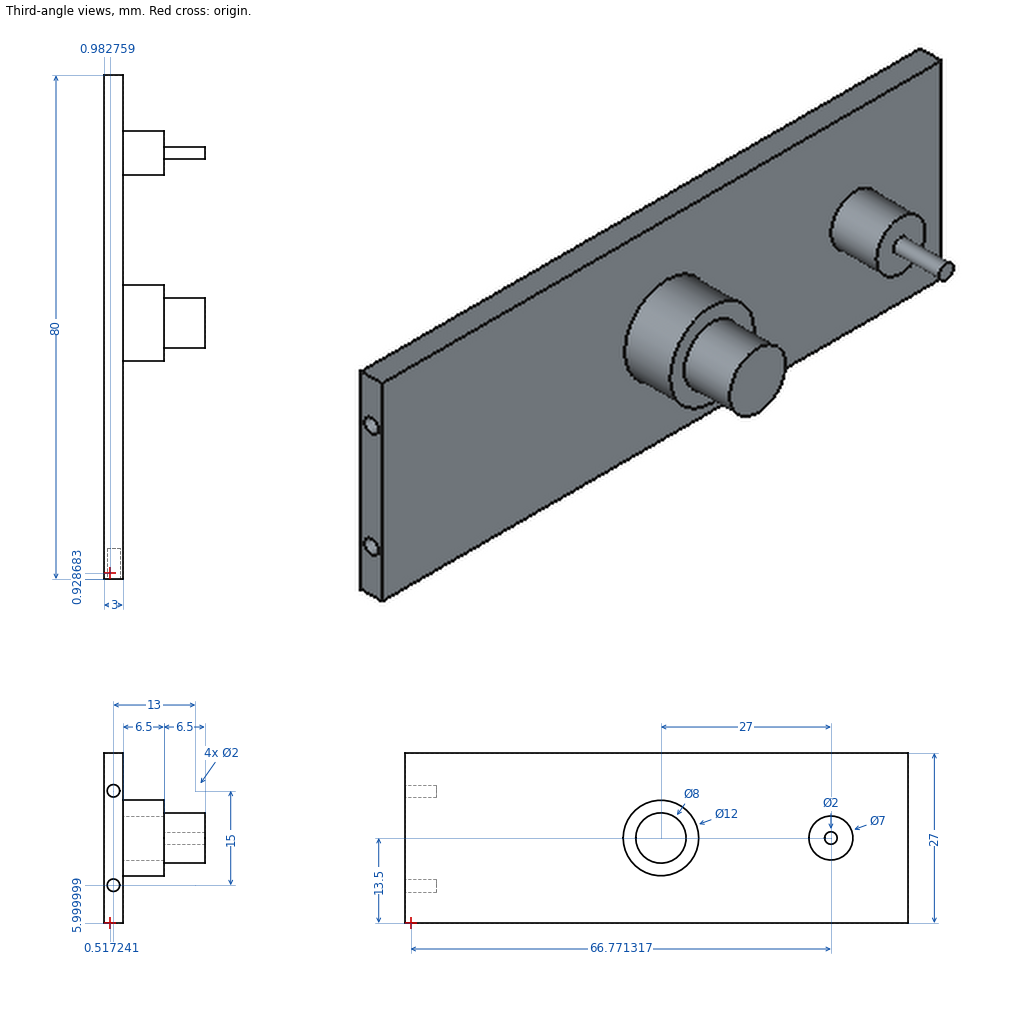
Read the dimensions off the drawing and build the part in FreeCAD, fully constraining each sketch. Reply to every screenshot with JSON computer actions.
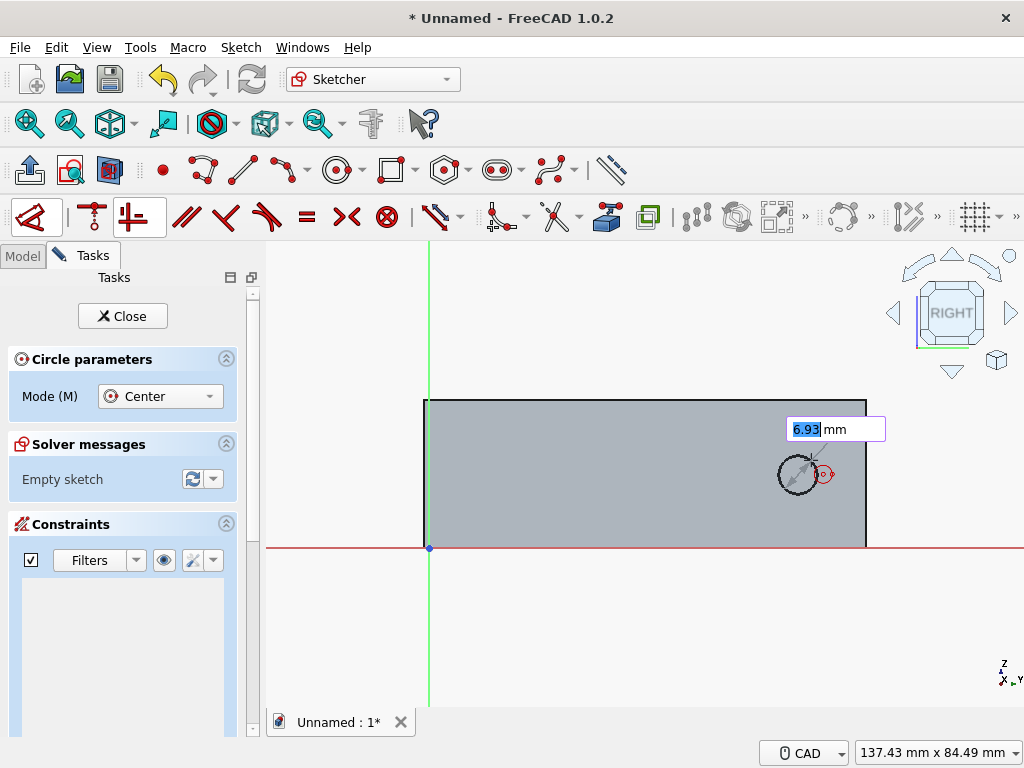
{"action": "type", "text": "7"}
{"action": "key", "text": "Return"}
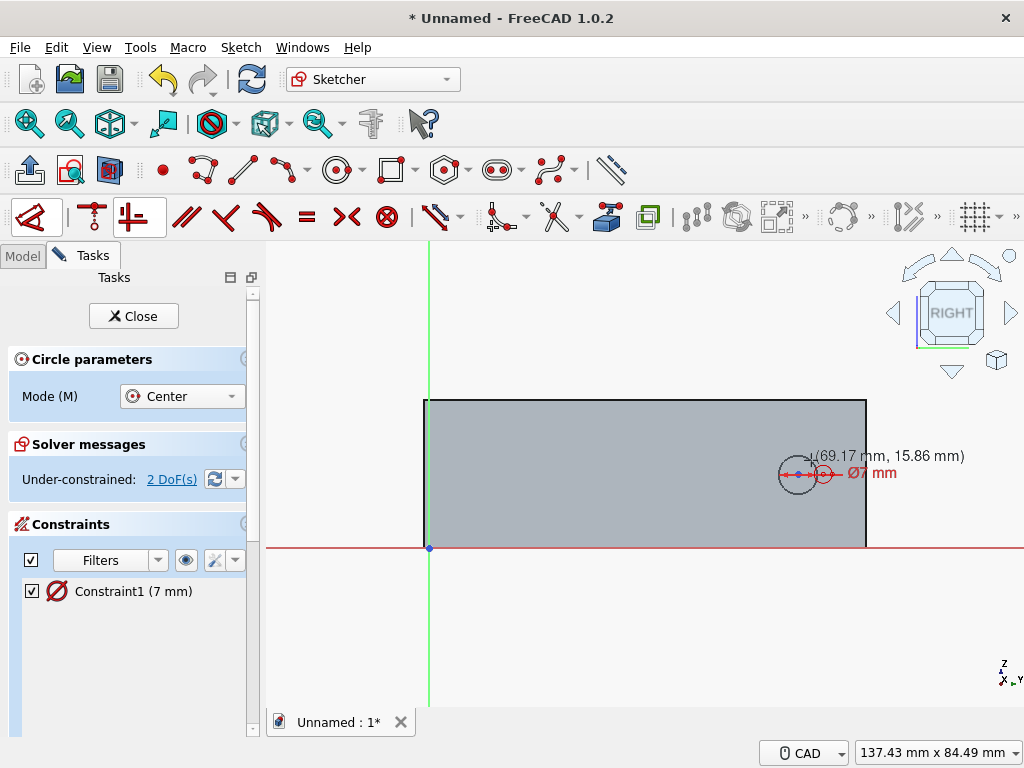
{"action": "left_click", "coordinate": [649, 474]}
{"action": "mouse_move", "coordinate": [672, 451]}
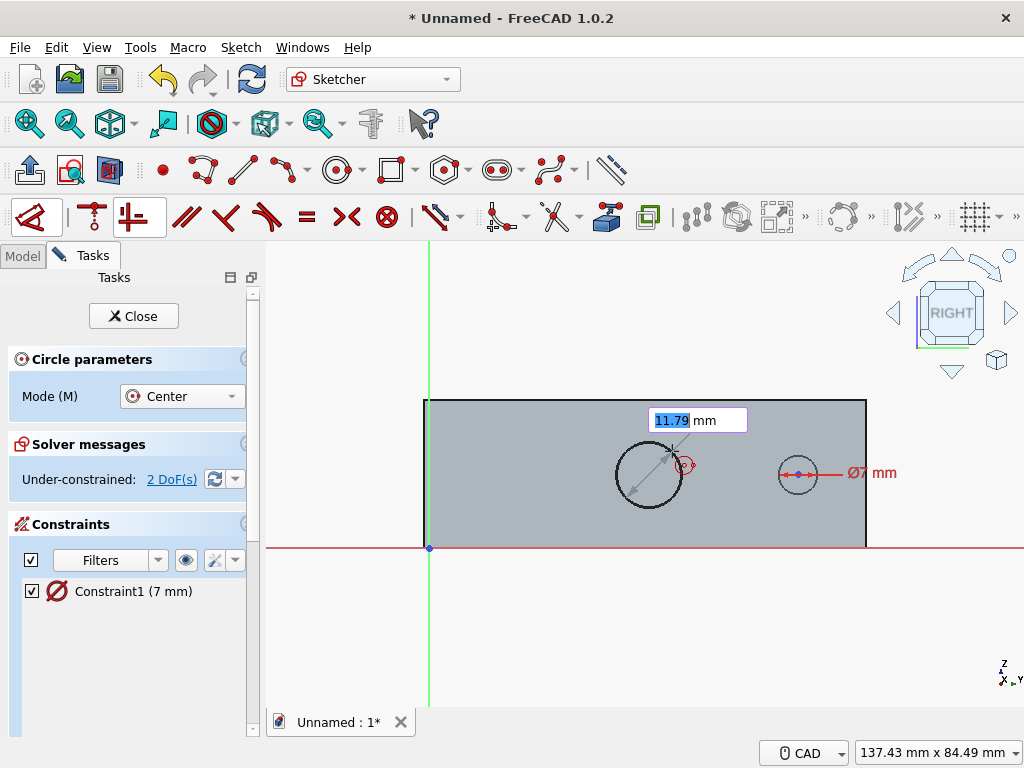
{"action": "type", "text": "12"}
{"action": "key", "text": "Return"}
{"action": "key", "text": "Escape"}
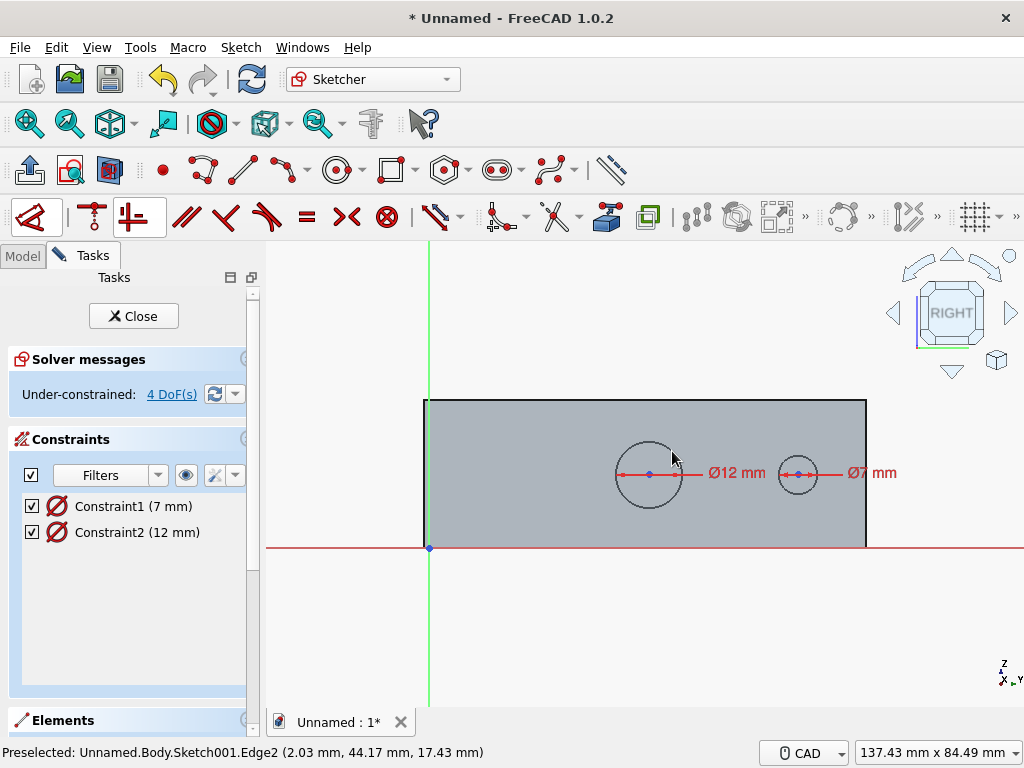
{"action": "left_click", "coordinate": [798, 475]}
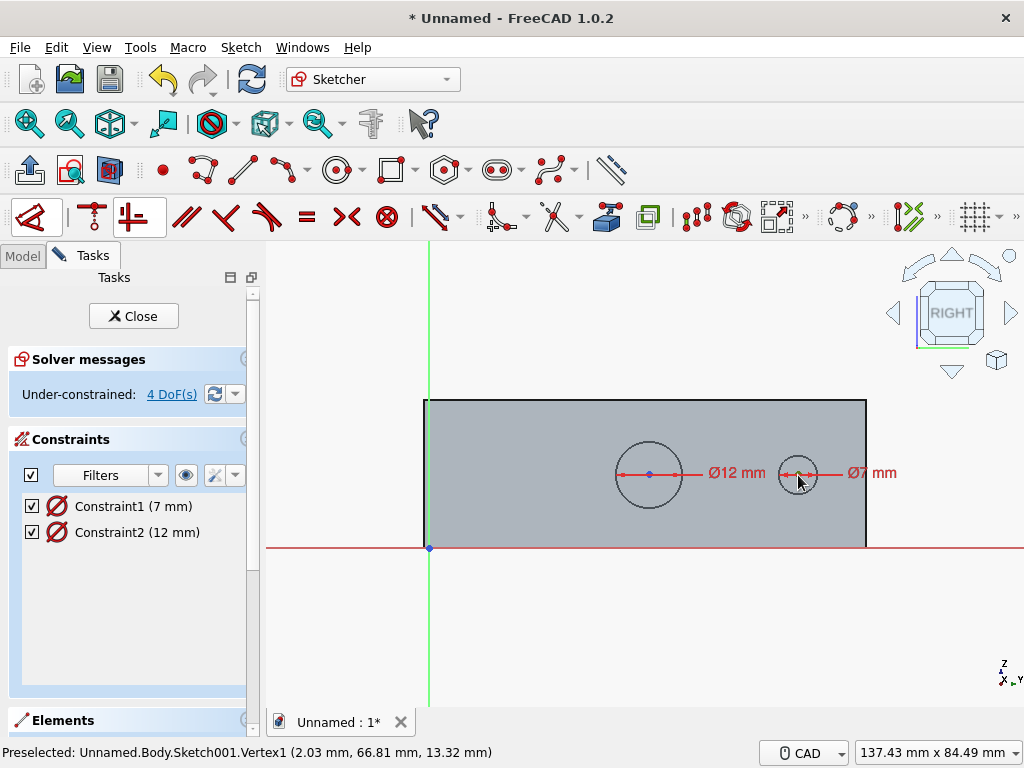
{"action": "left_click", "coordinate": [649, 475]}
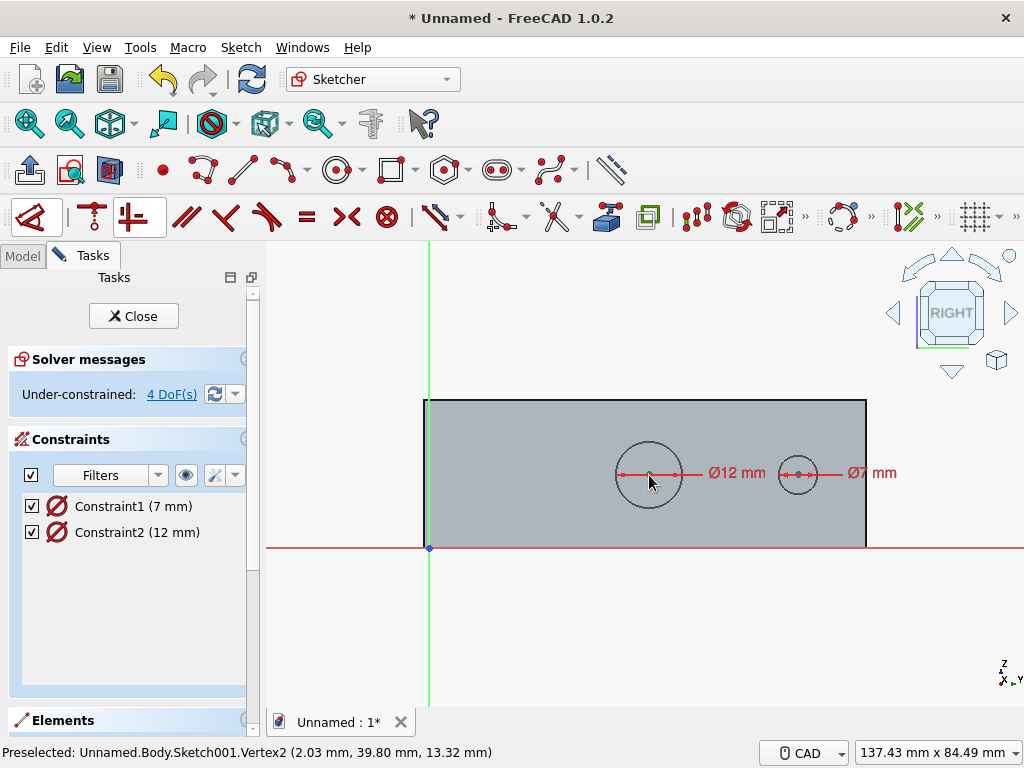
{"action": "left_click", "coordinate": [160, 218]}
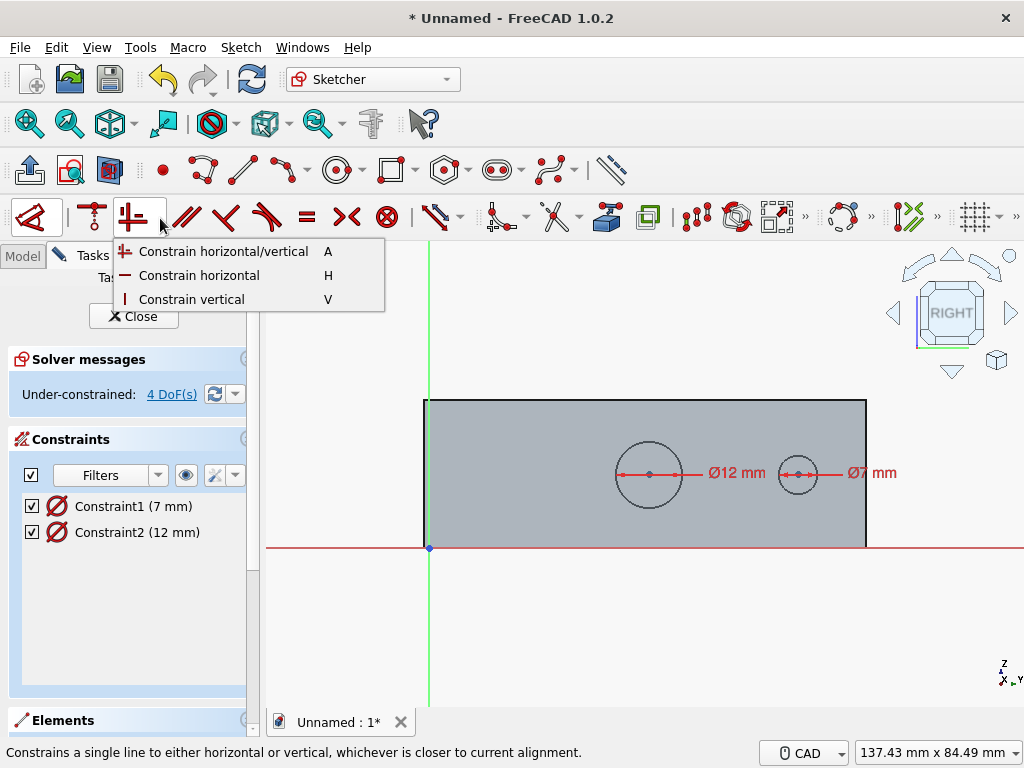
{"action": "left_click", "coordinate": [249, 275]}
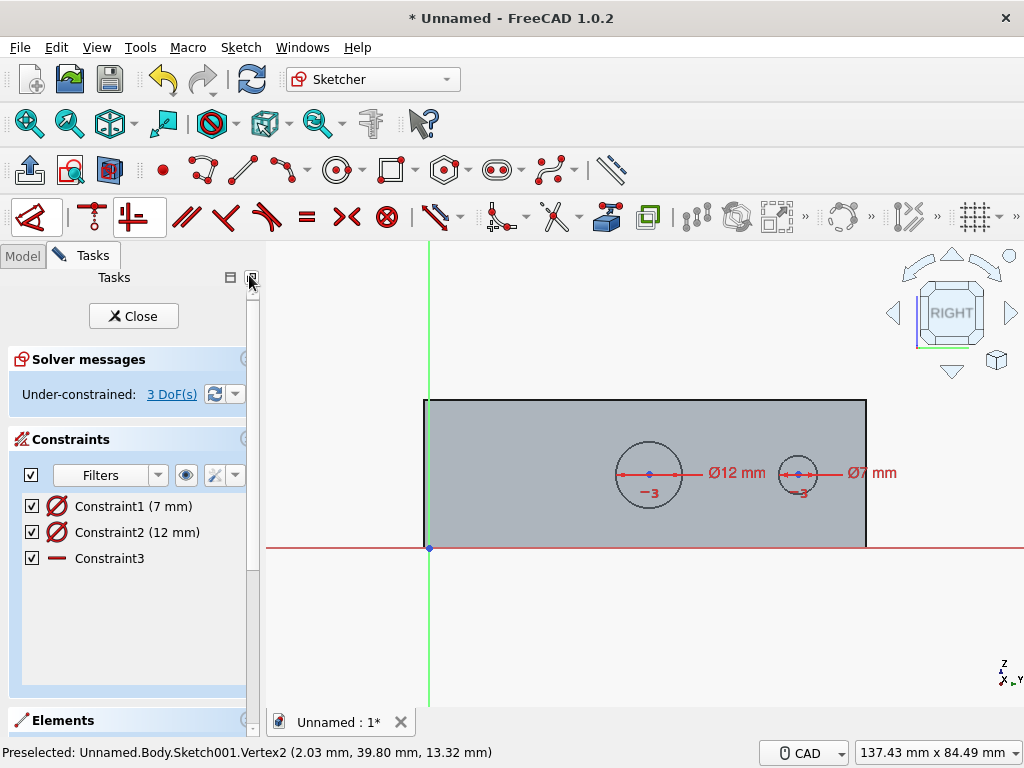
{"action": "left_click", "coordinate": [798, 475]}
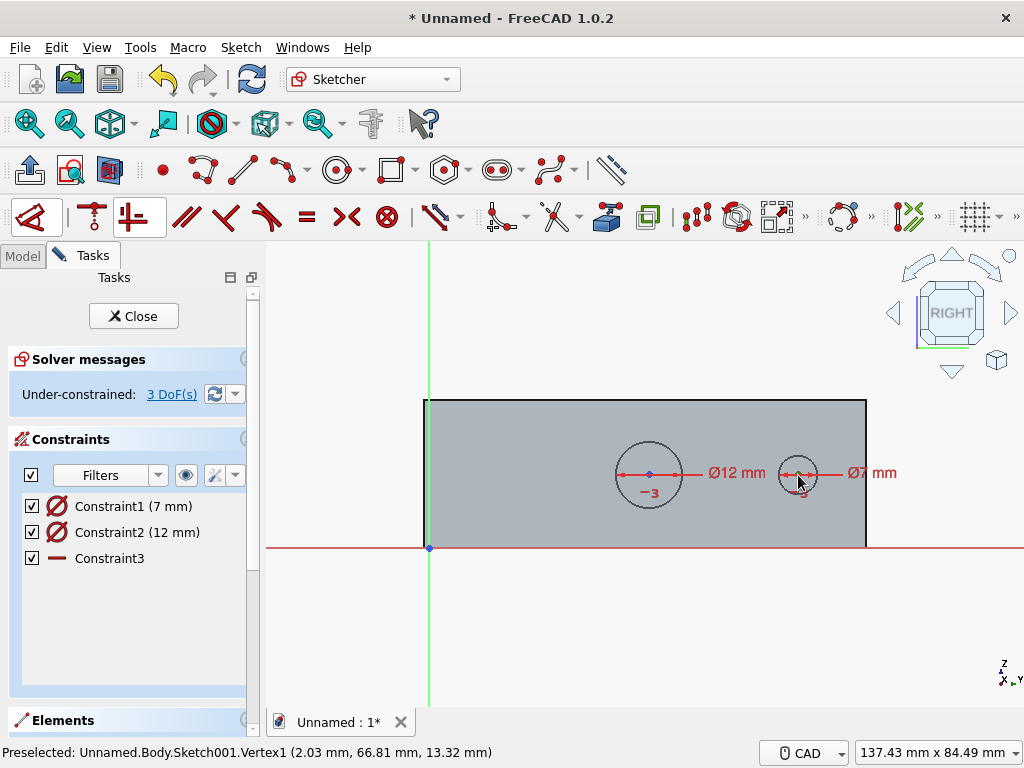
{"action": "left_click", "coordinate": [649, 475]}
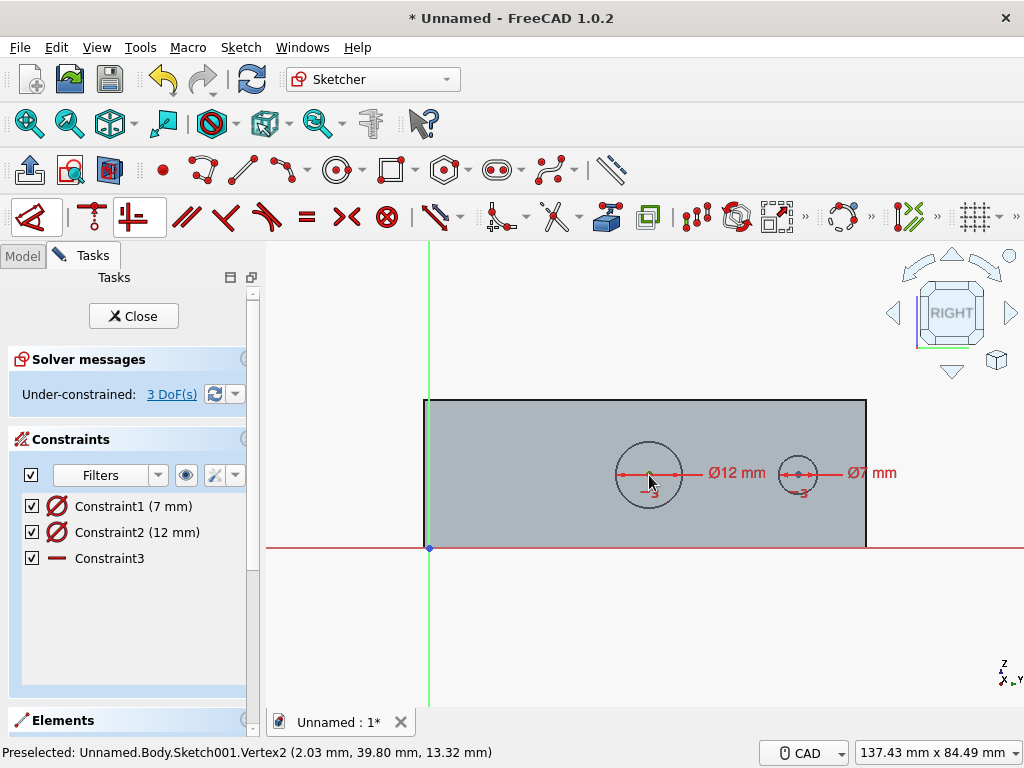
{"action": "key", "text": "l"}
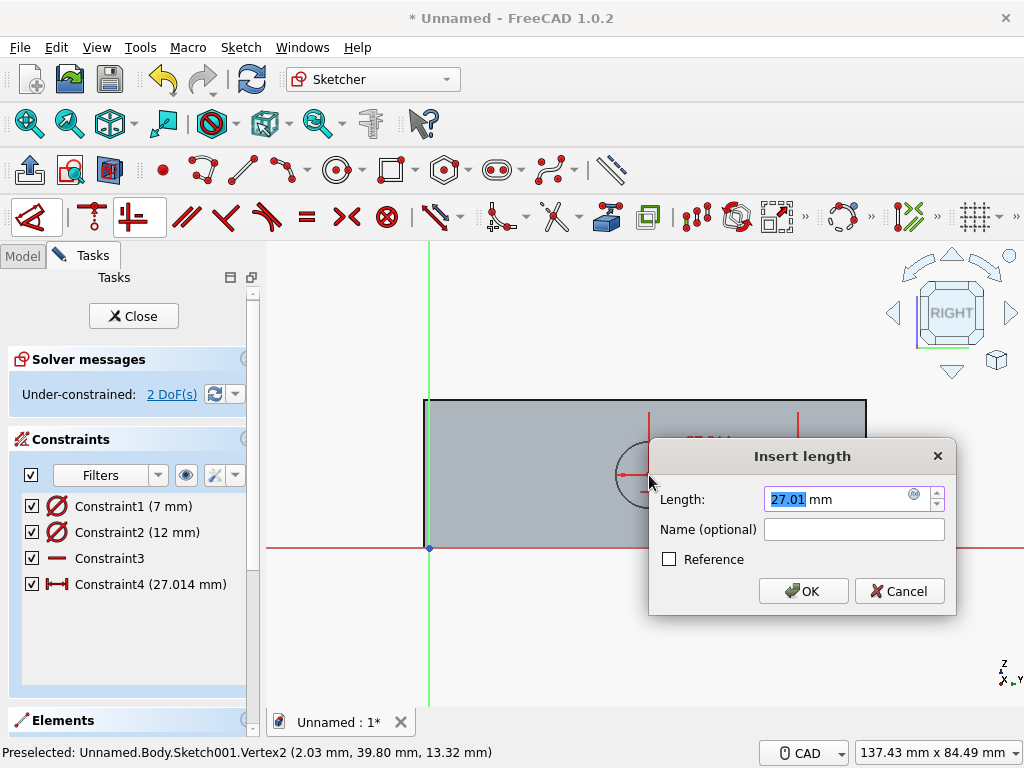
{"action": "type", "text": "27"}
{"action": "key", "text": "Return"}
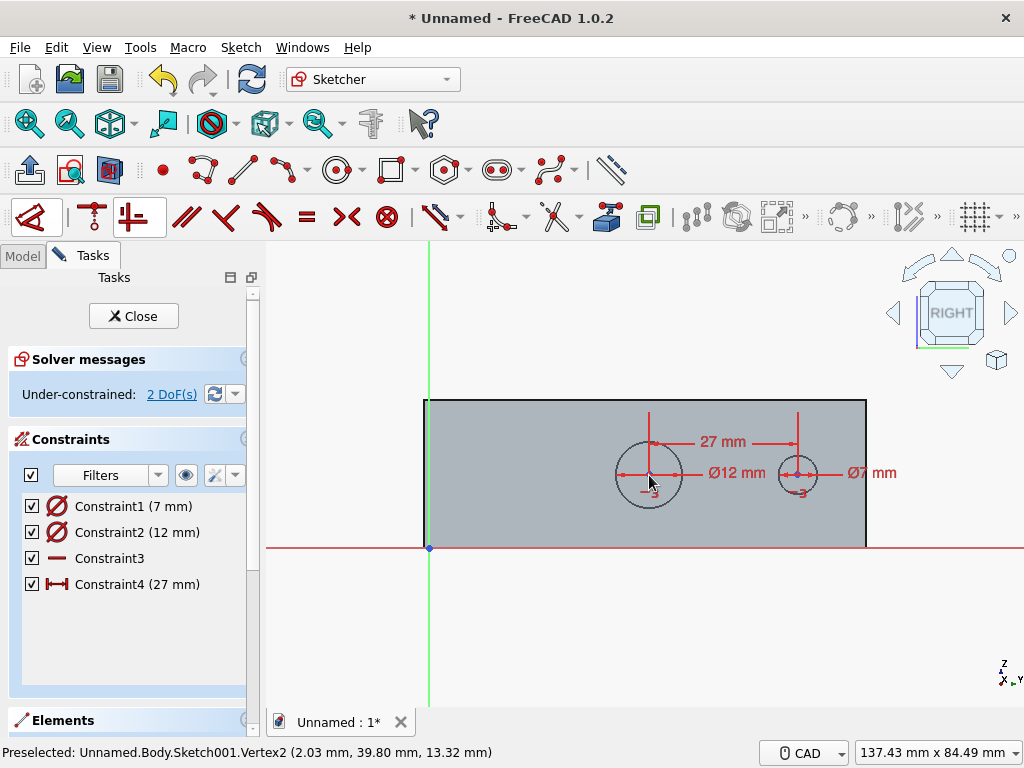
{"action": "left_click", "coordinate": [798, 475]}